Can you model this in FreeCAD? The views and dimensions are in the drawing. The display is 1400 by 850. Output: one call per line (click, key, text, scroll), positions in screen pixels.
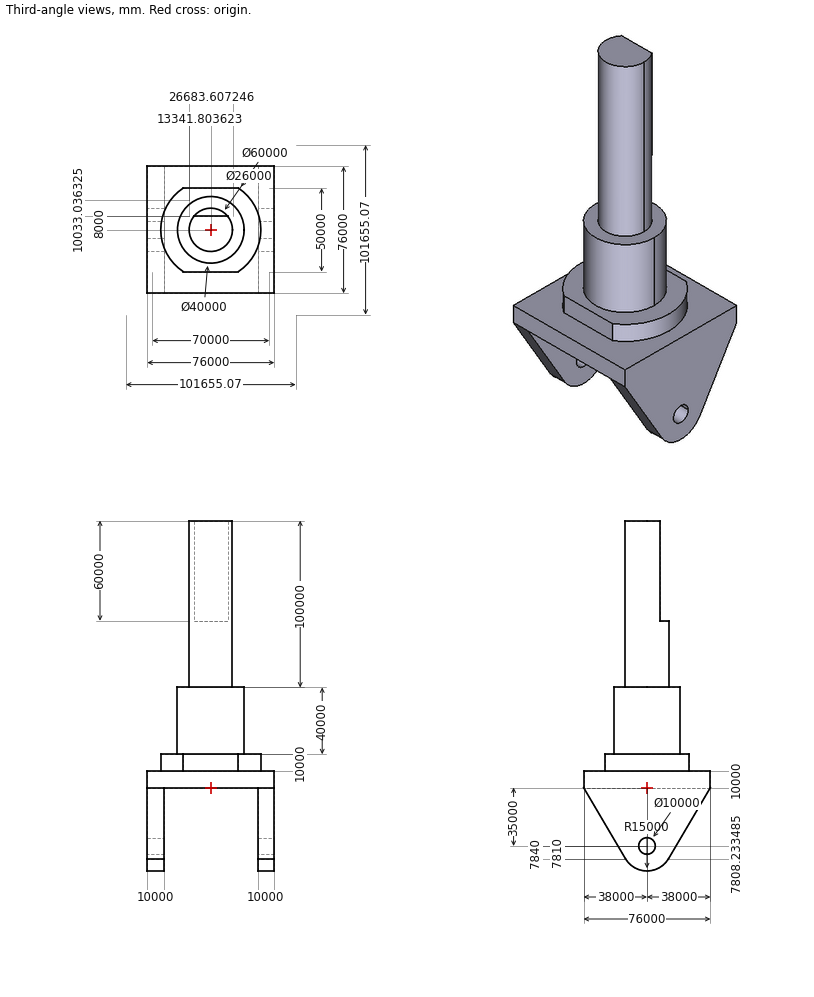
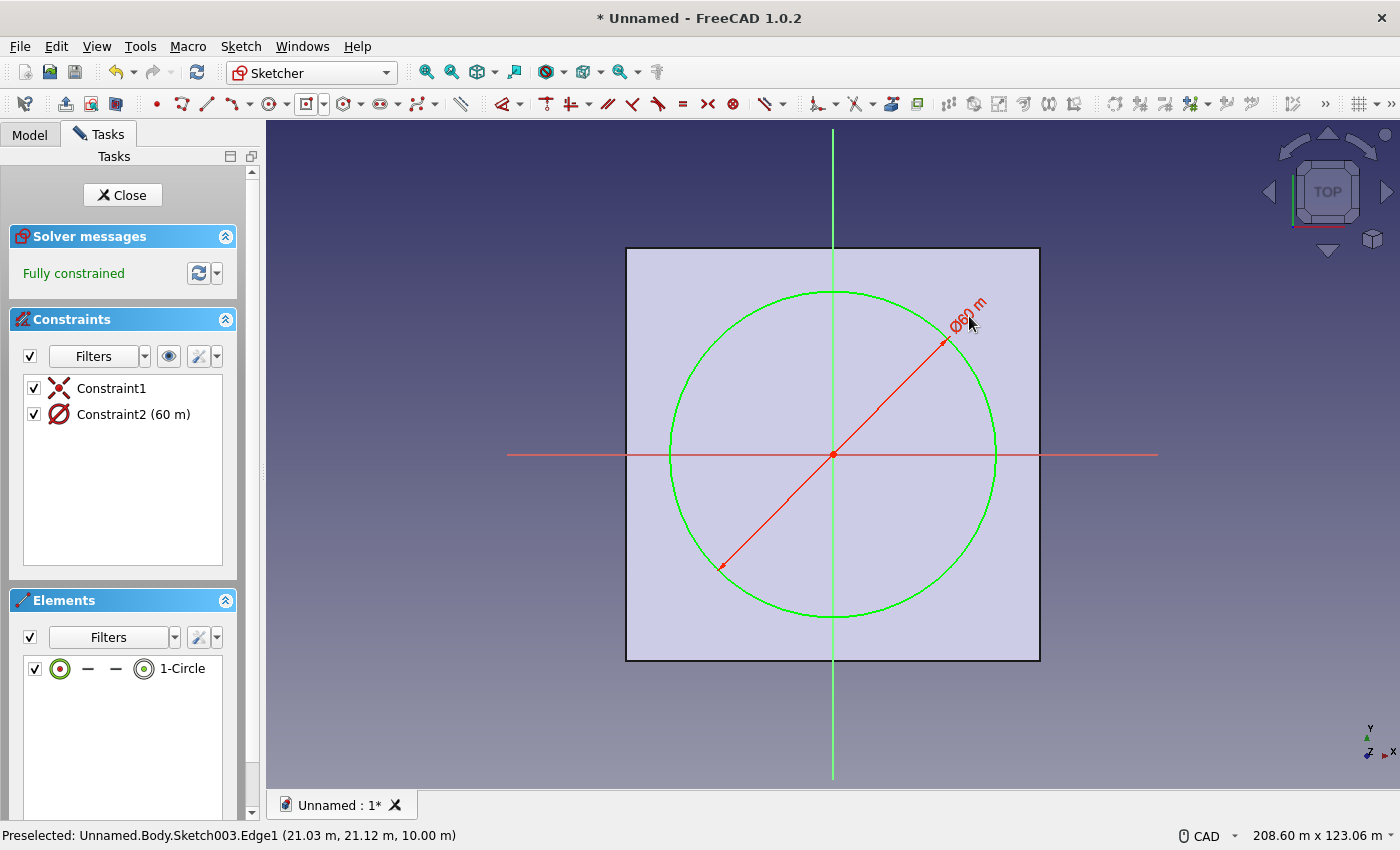
click(123, 195)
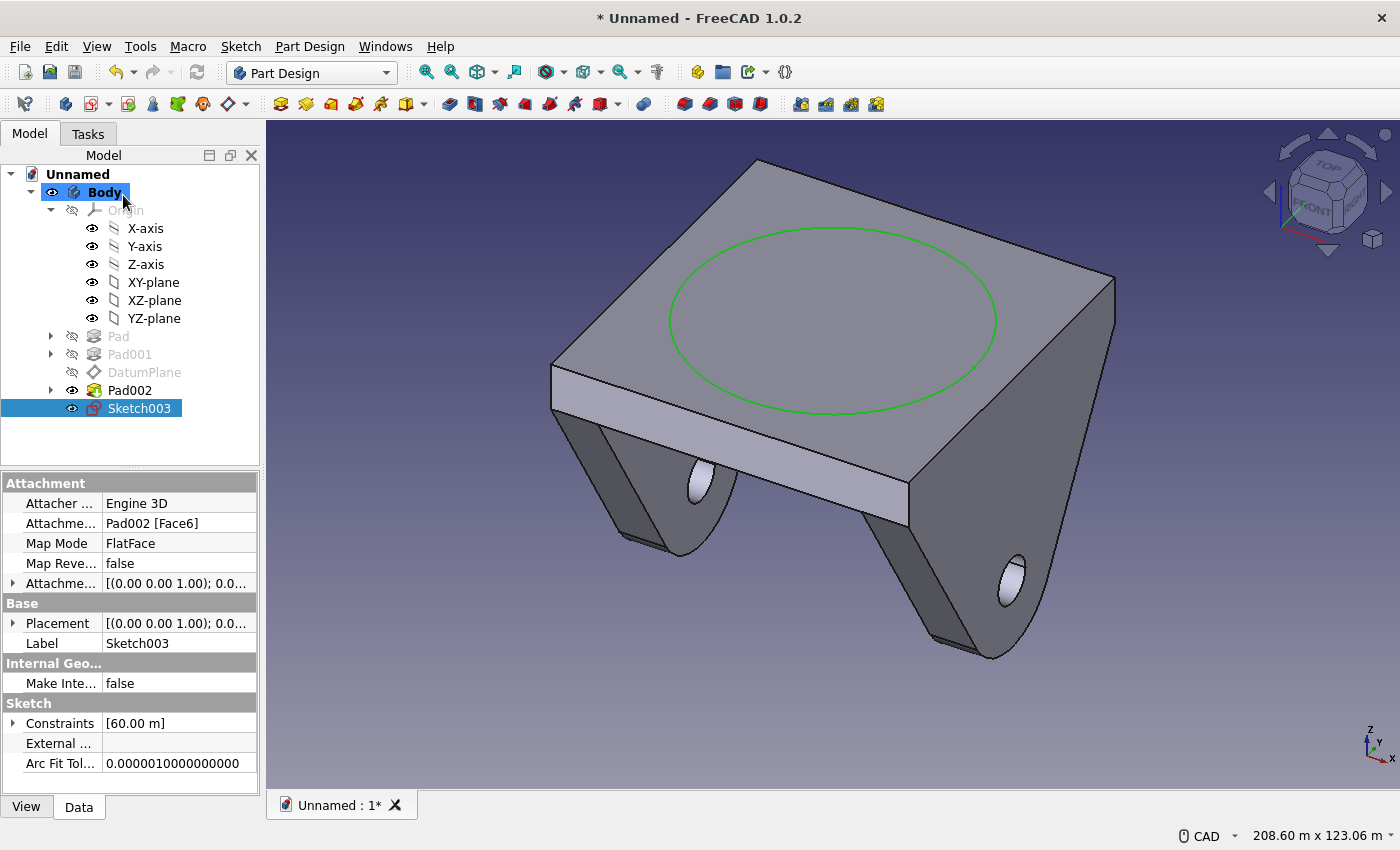
click(281, 104)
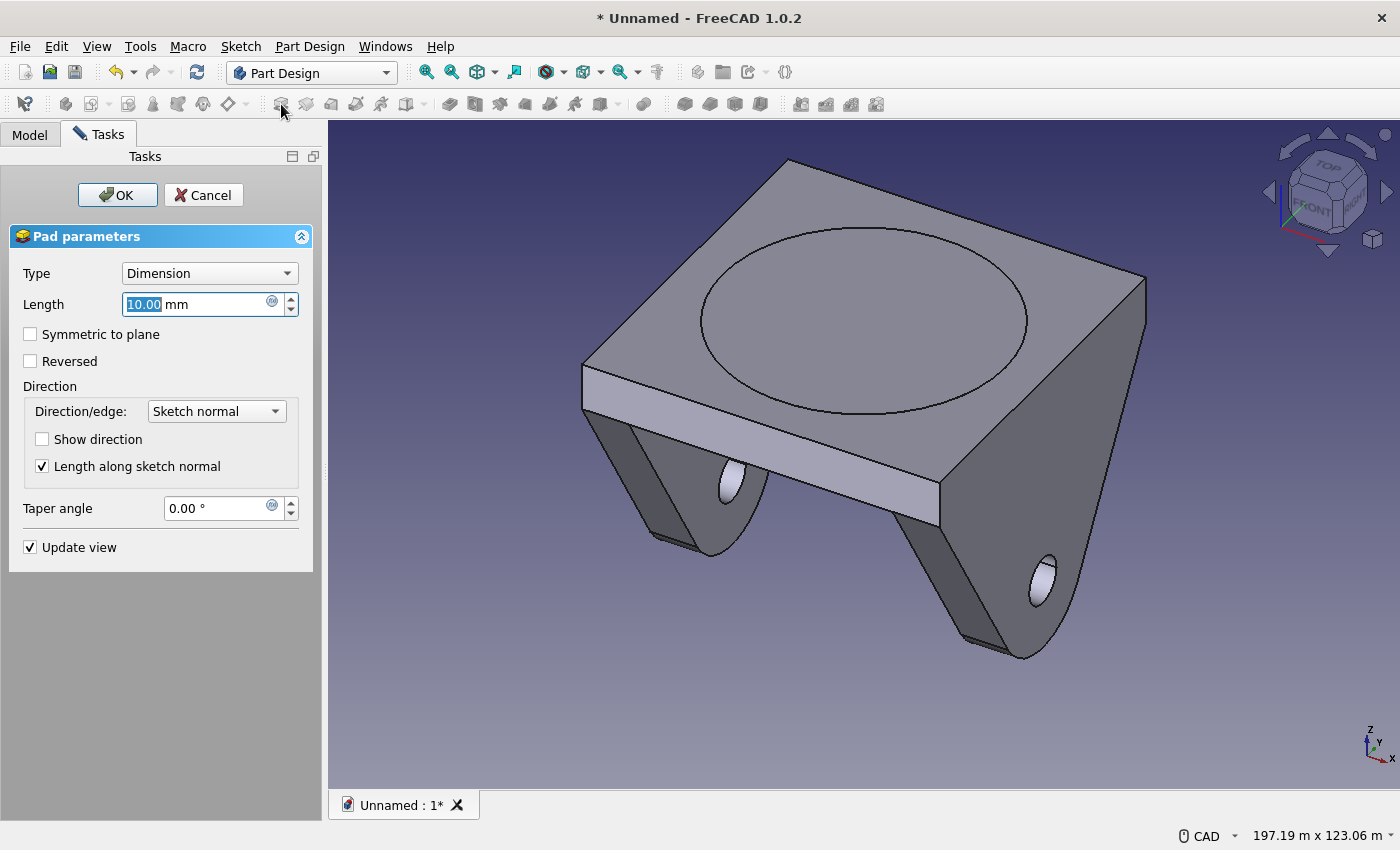
text(10000)
key(Tab)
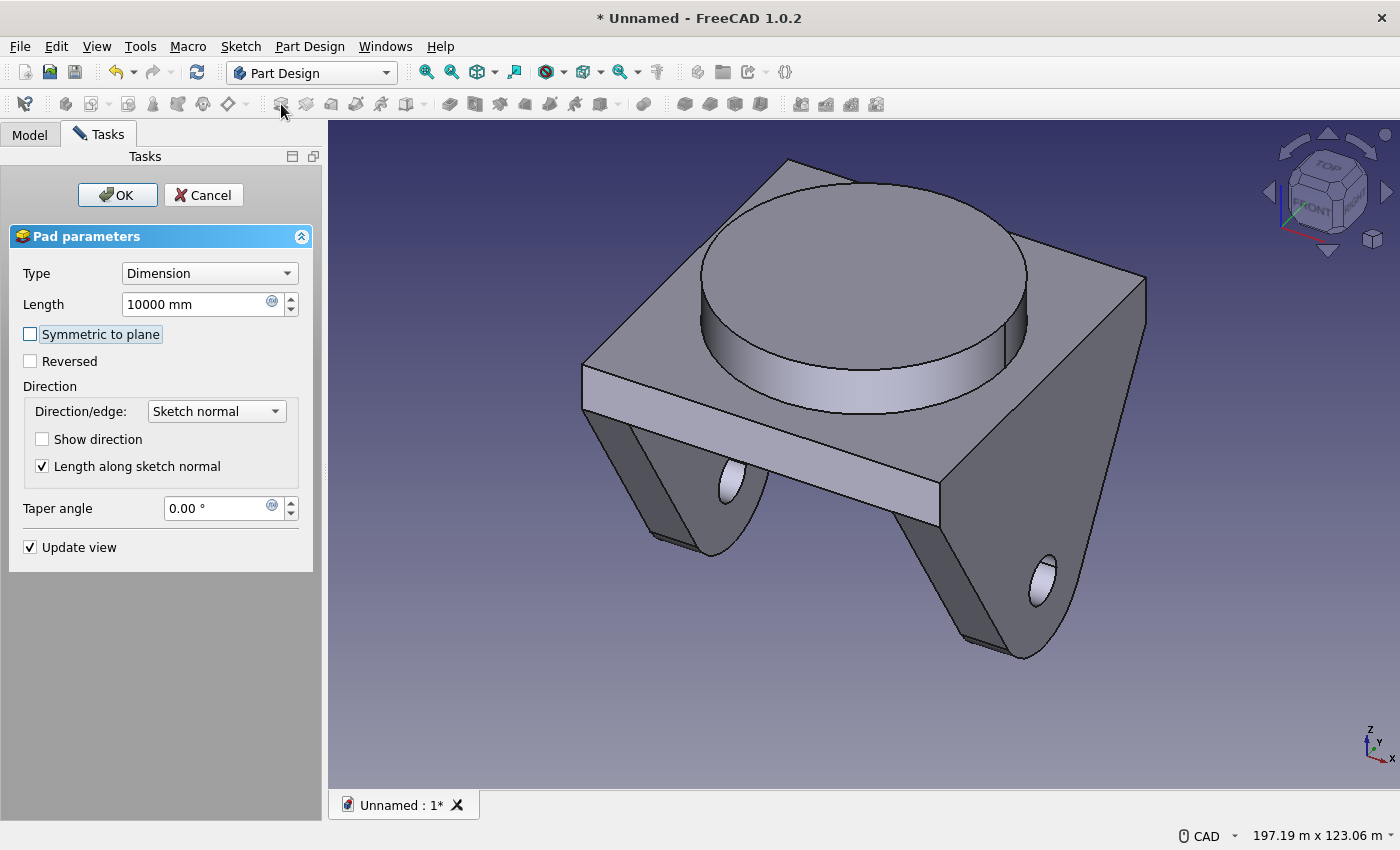
click(118, 195)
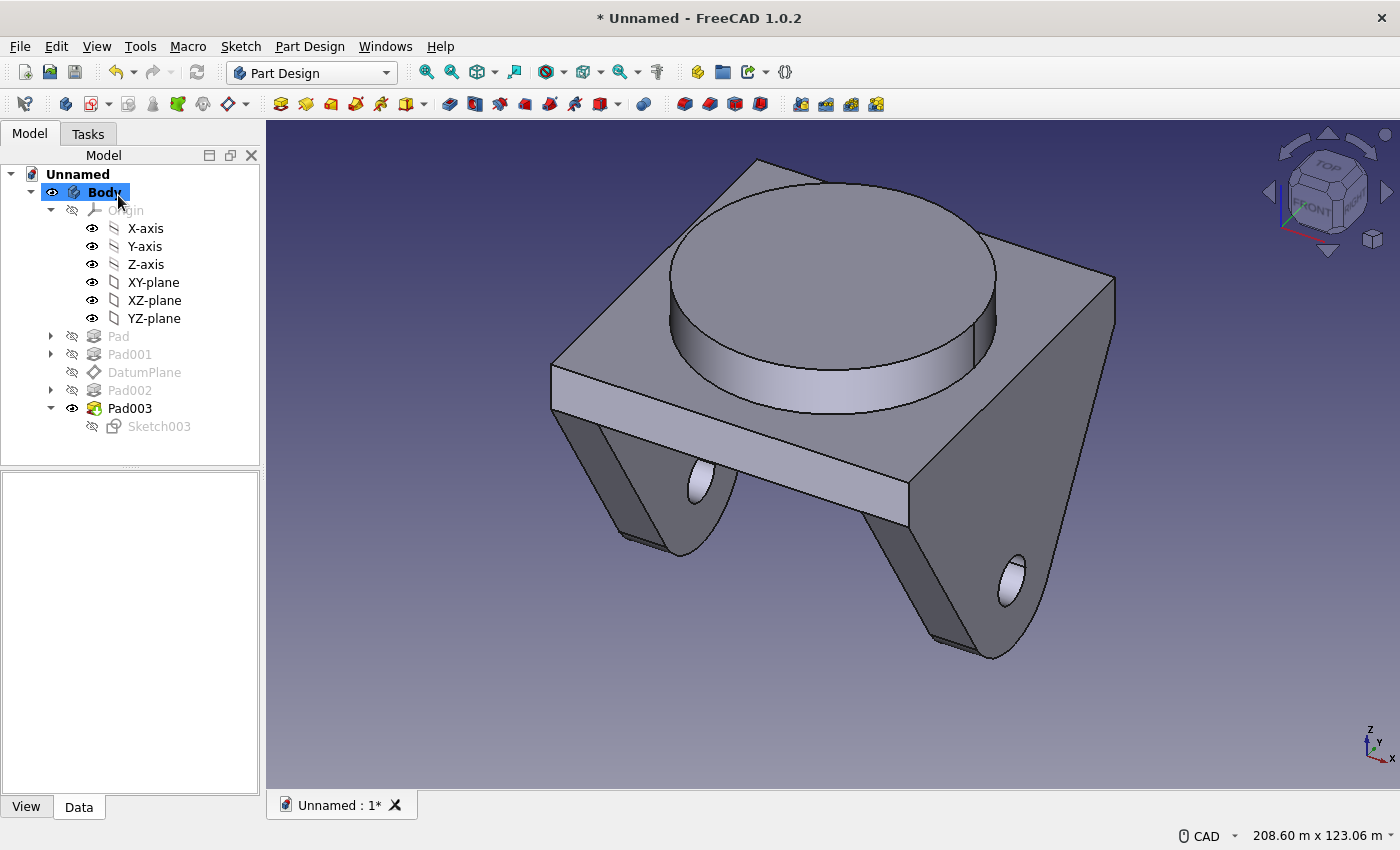
key(v)
key(f)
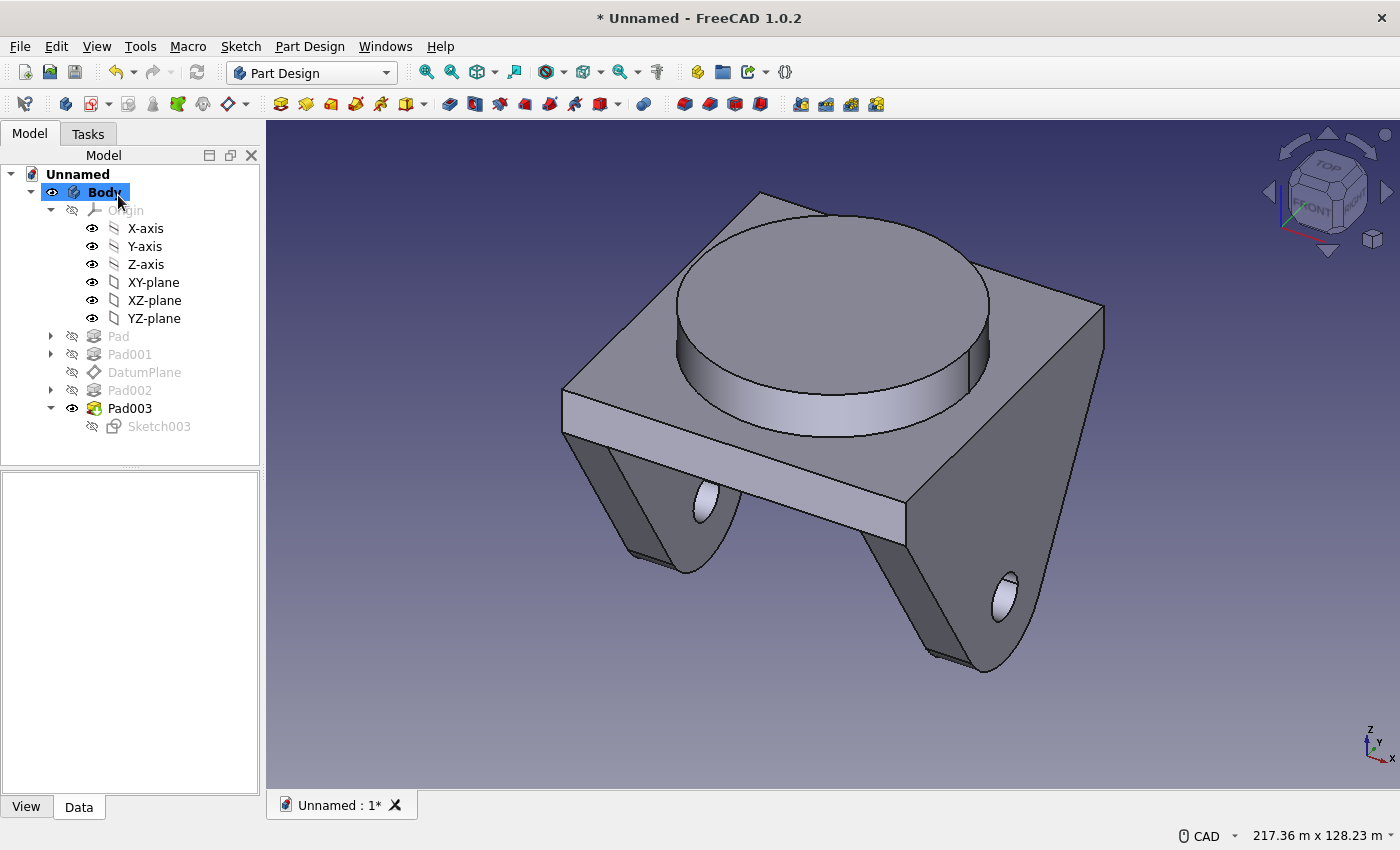
click(833, 304)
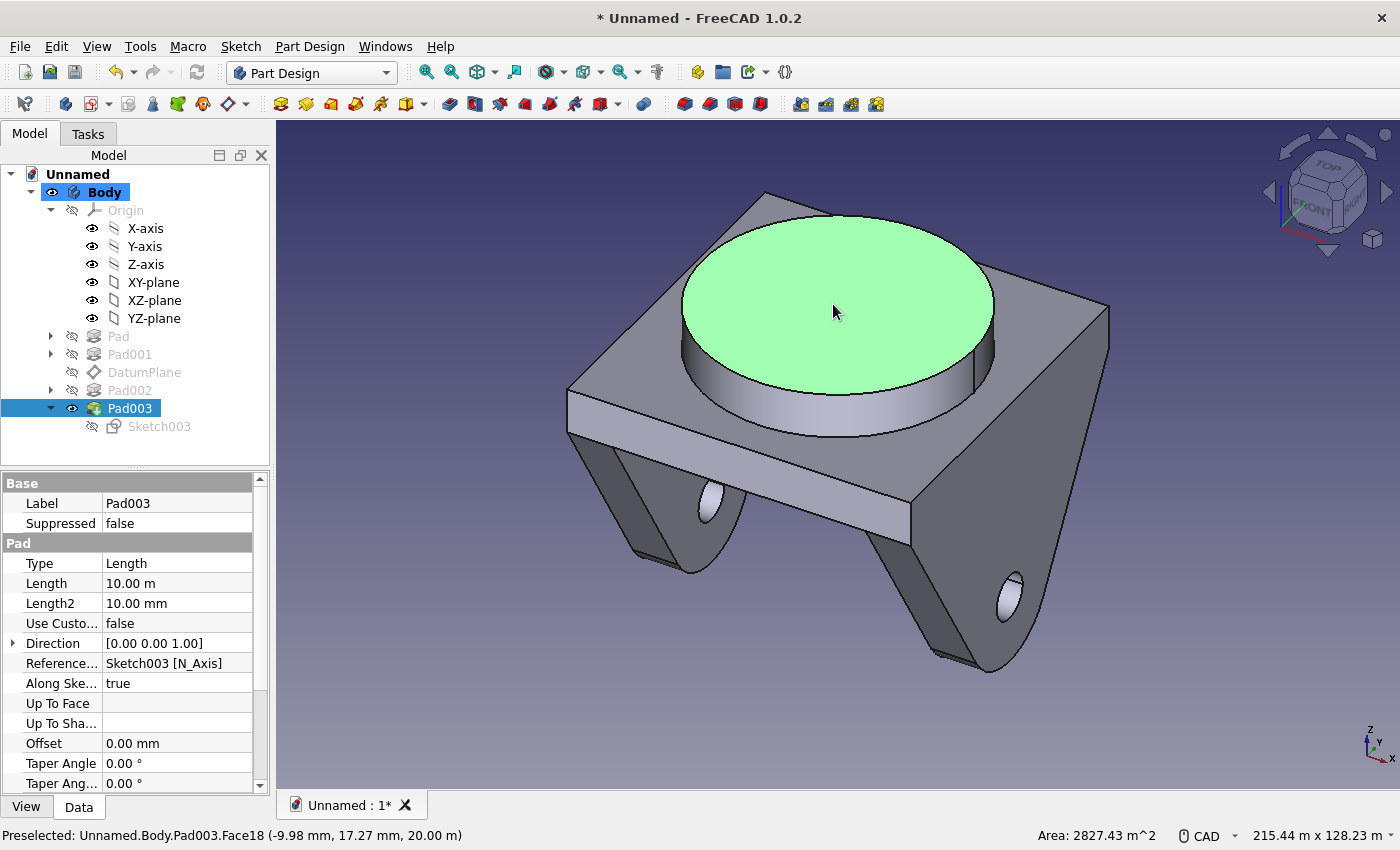
click(90, 104)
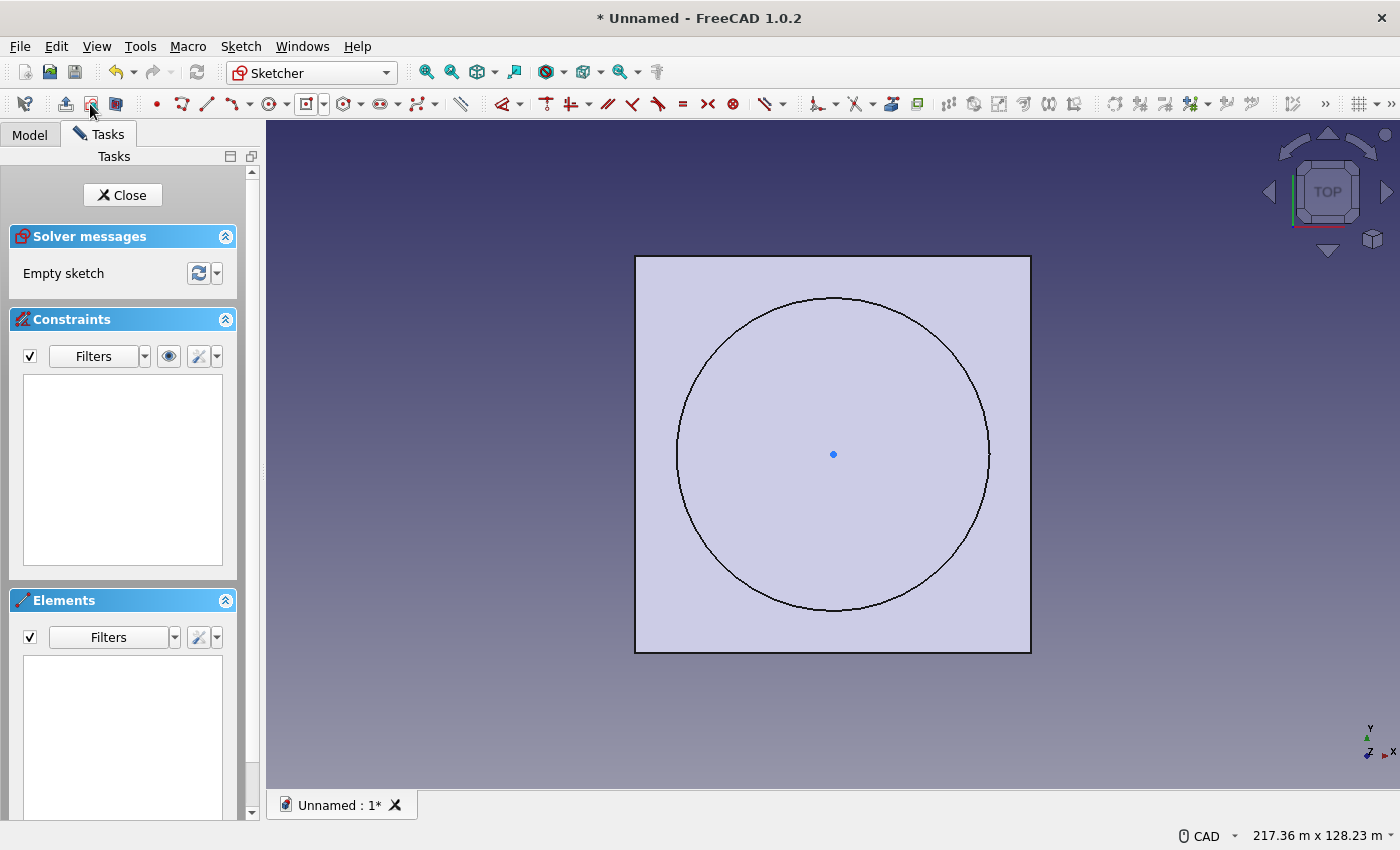
click(306, 104)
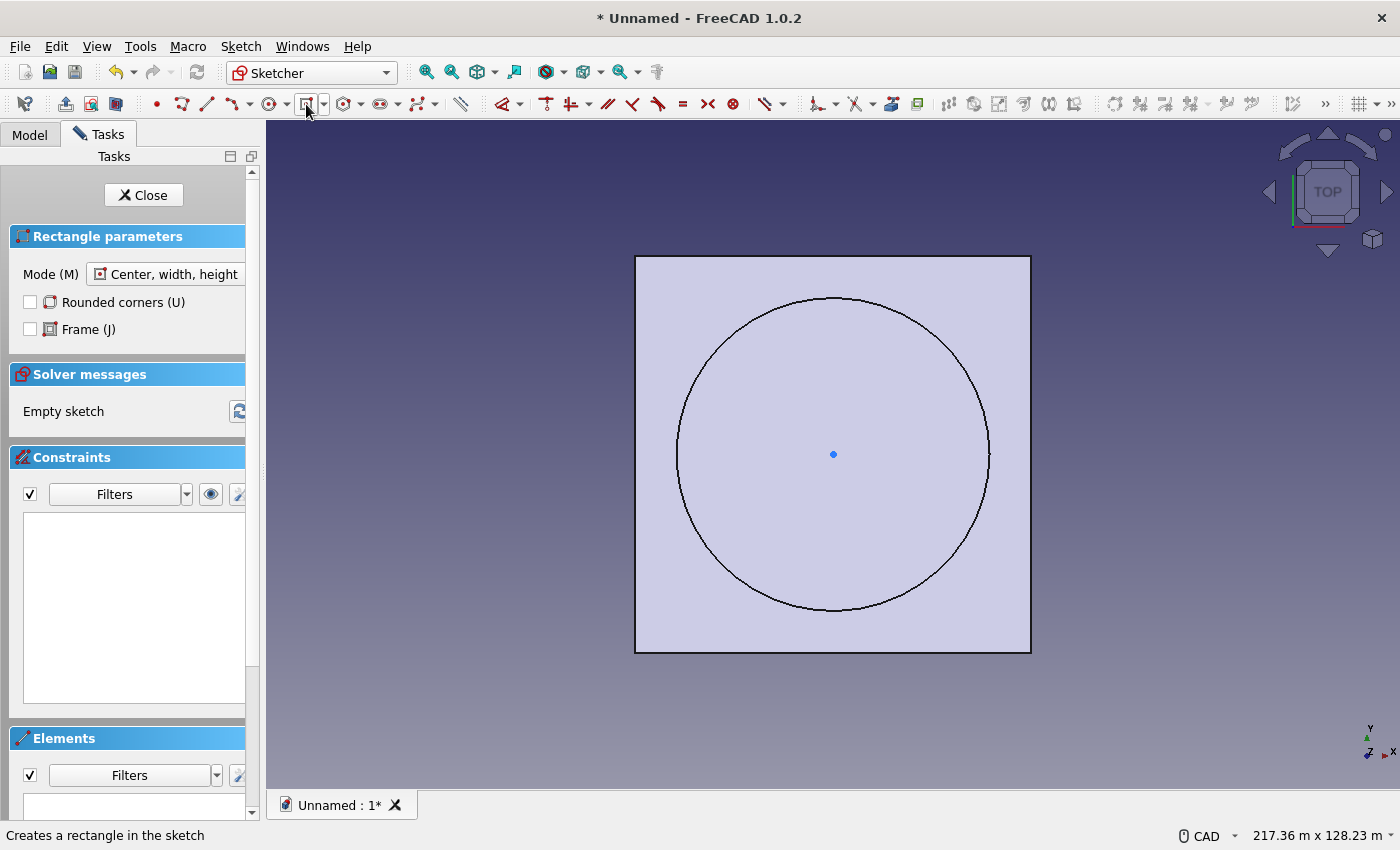
click(833, 454)
click(1098, 189)